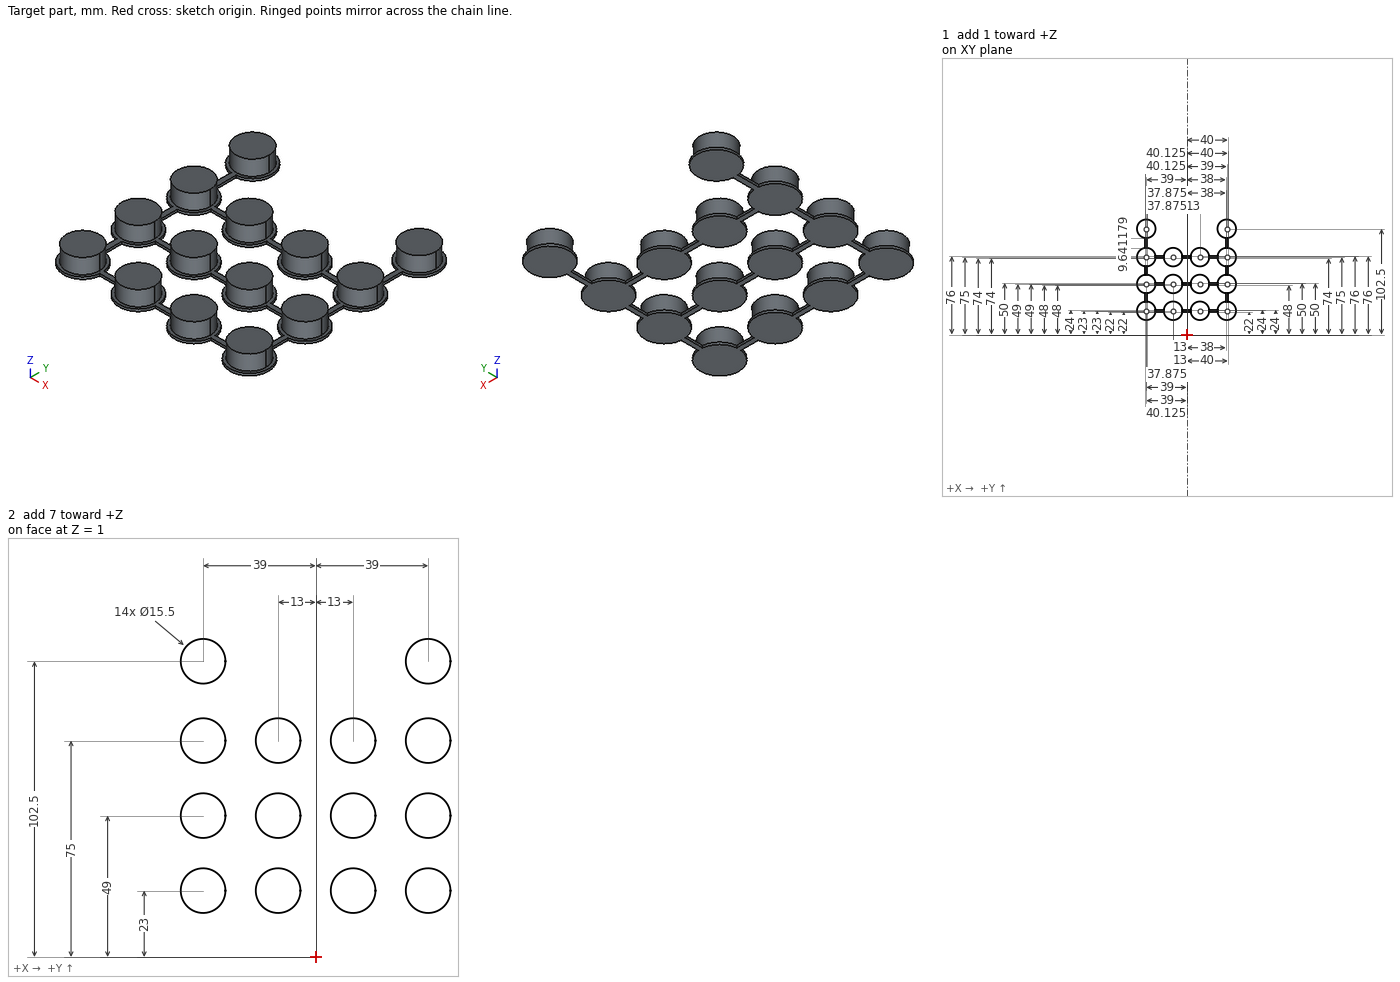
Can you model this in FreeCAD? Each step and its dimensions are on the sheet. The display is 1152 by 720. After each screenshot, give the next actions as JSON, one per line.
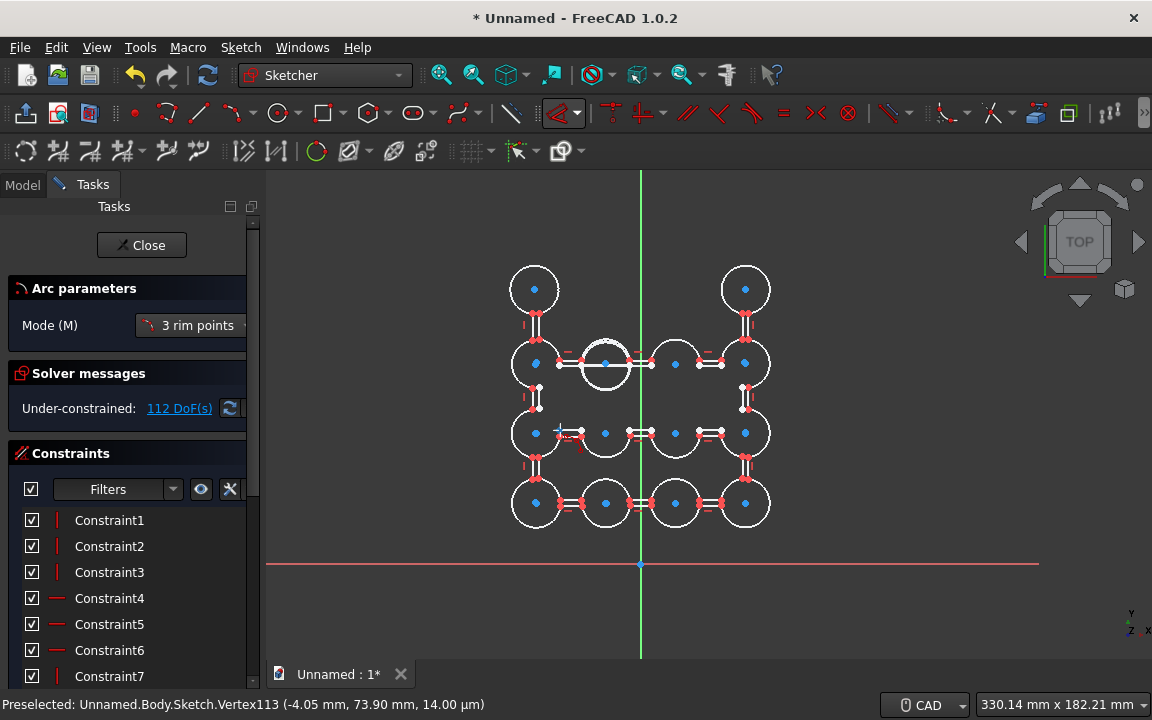
{"action": "left_click", "coordinate": [606, 387]}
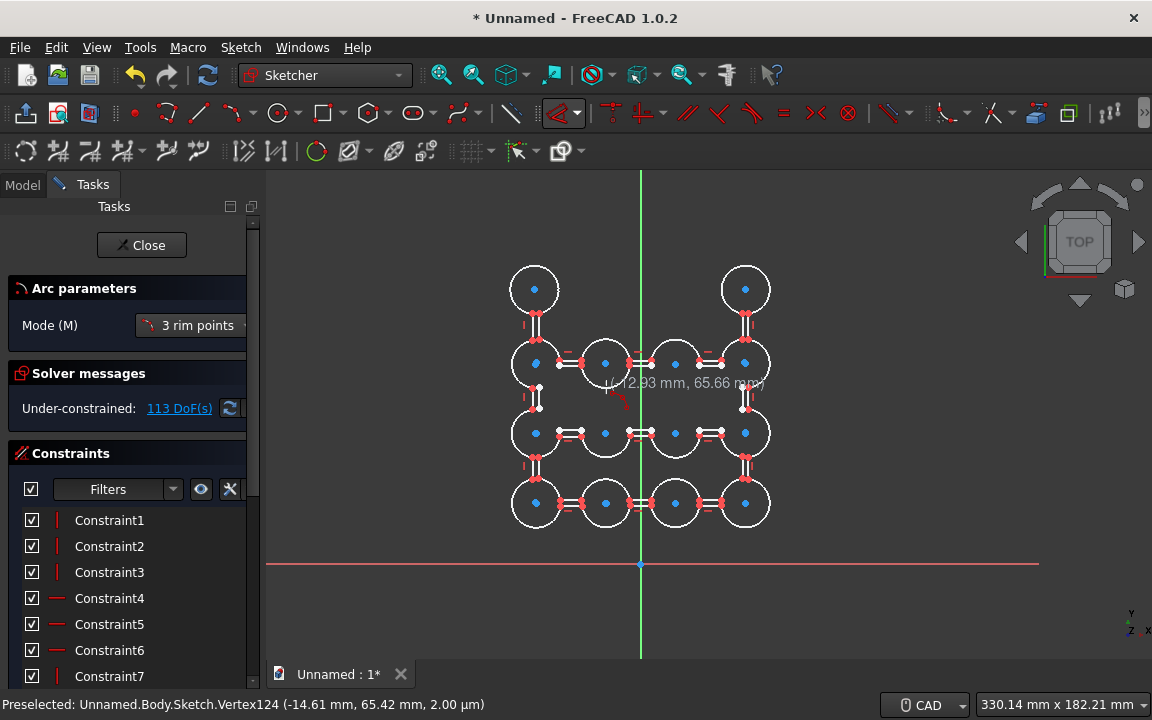
{"action": "scroll", "coordinate": [652, 366], "scroll_direction": "up", "scroll_amount": 6}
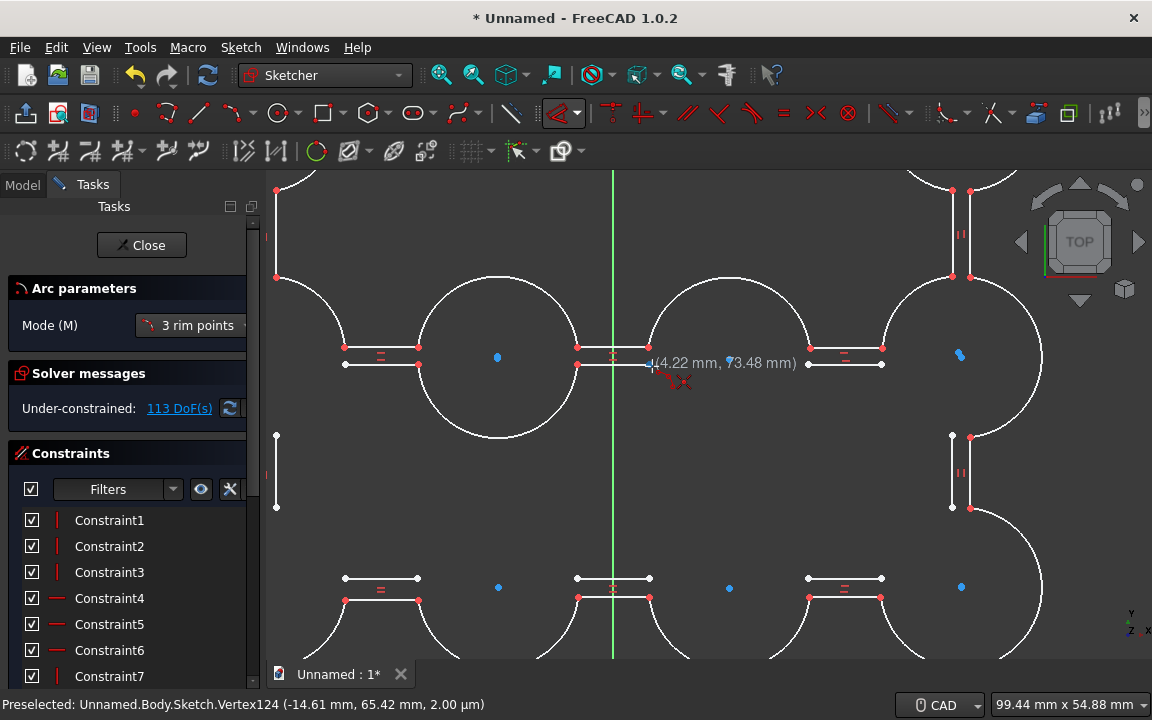
{"action": "left_click", "coordinate": [649, 365]}
{"action": "left_click", "coordinate": [808, 365]}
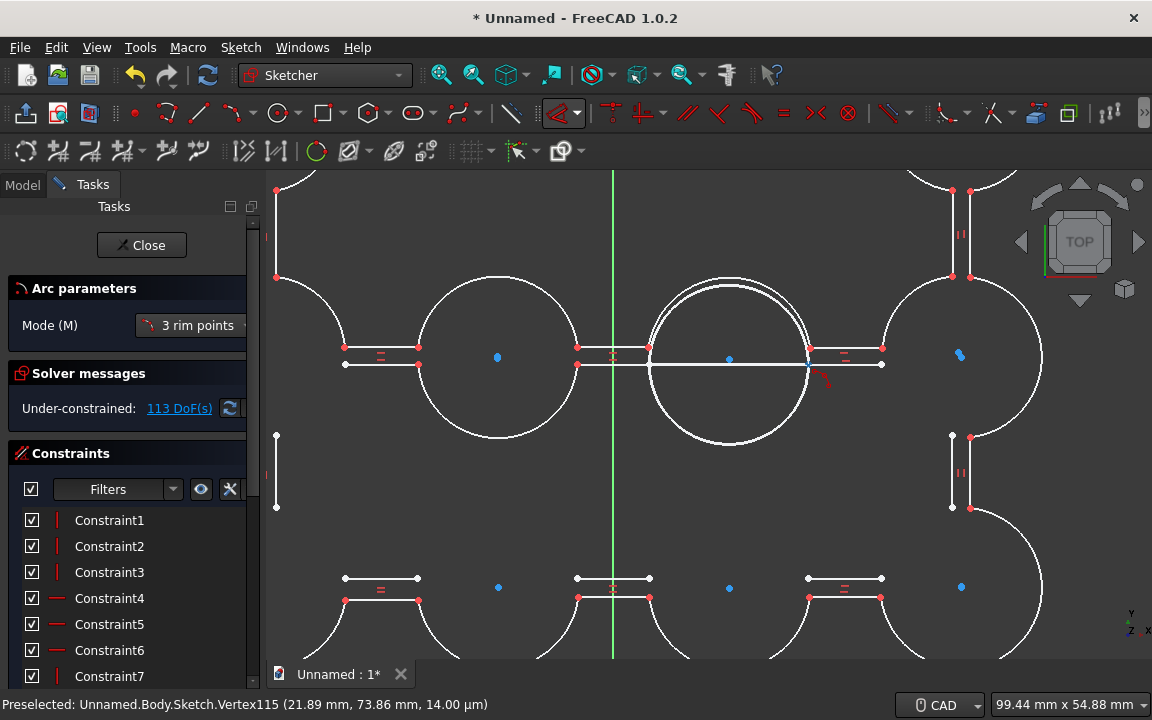
{"action": "scroll", "coordinate": [652, 366], "scroll_direction": "down", "scroll_amount": 6}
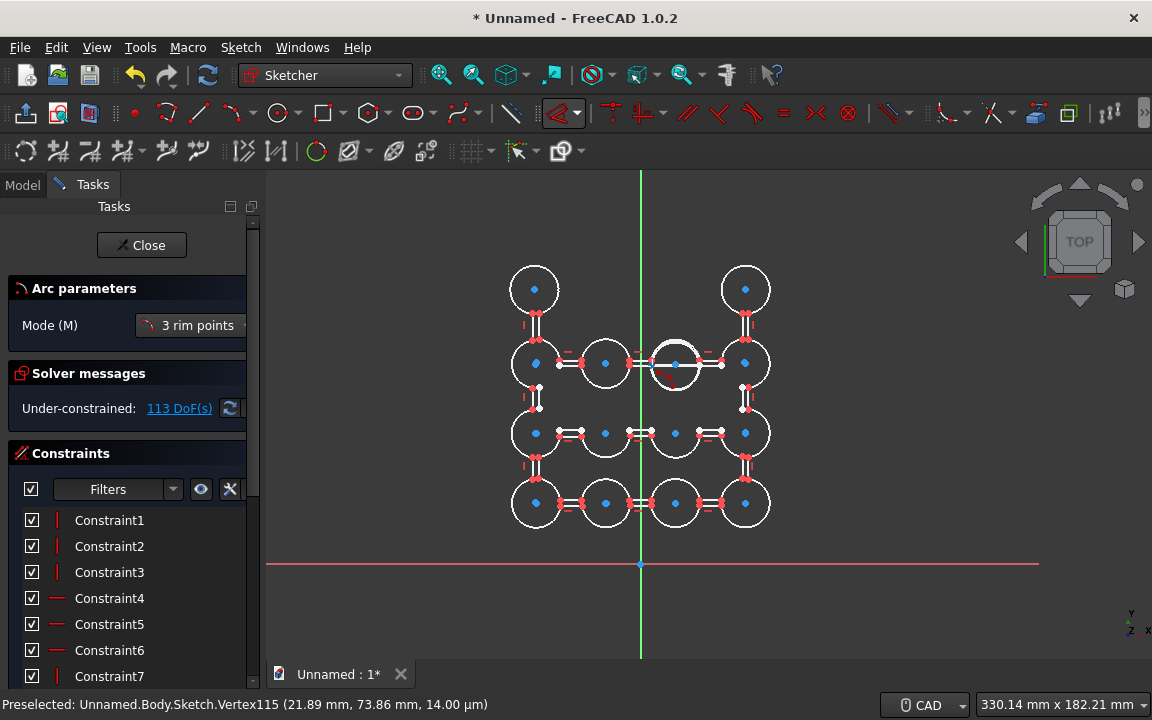
{"action": "left_click", "coordinate": [676, 387]}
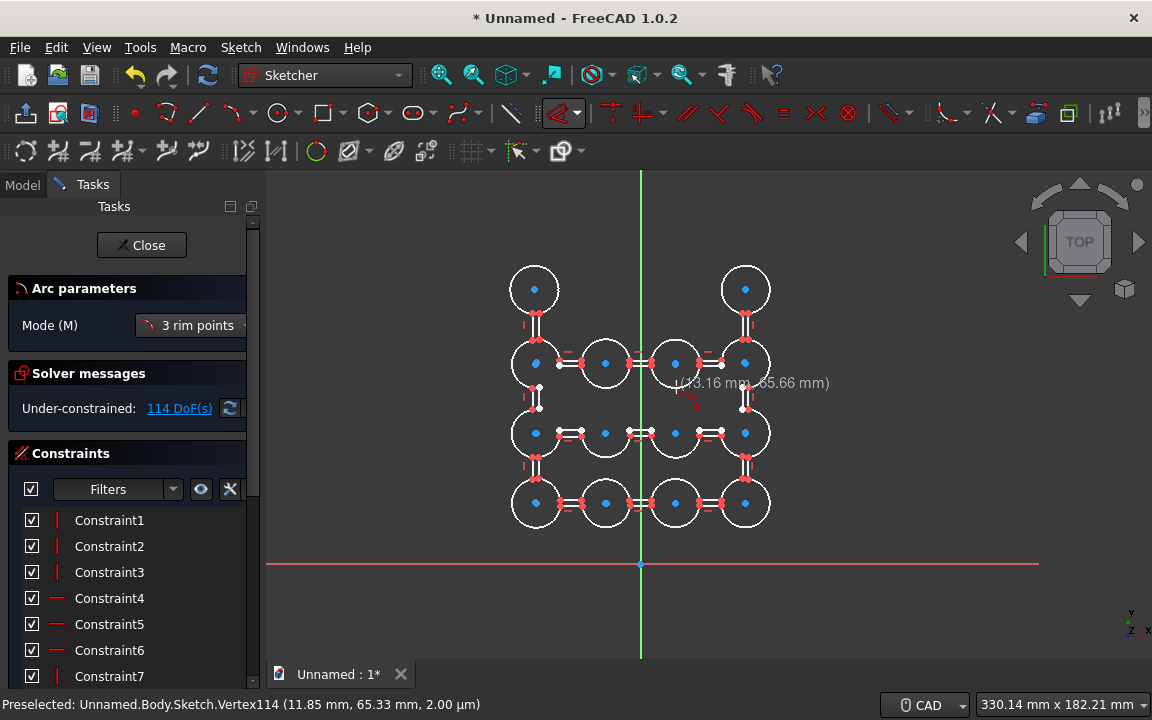
{"action": "scroll", "coordinate": [721, 366], "scroll_direction": "up", "scroll_amount": 6}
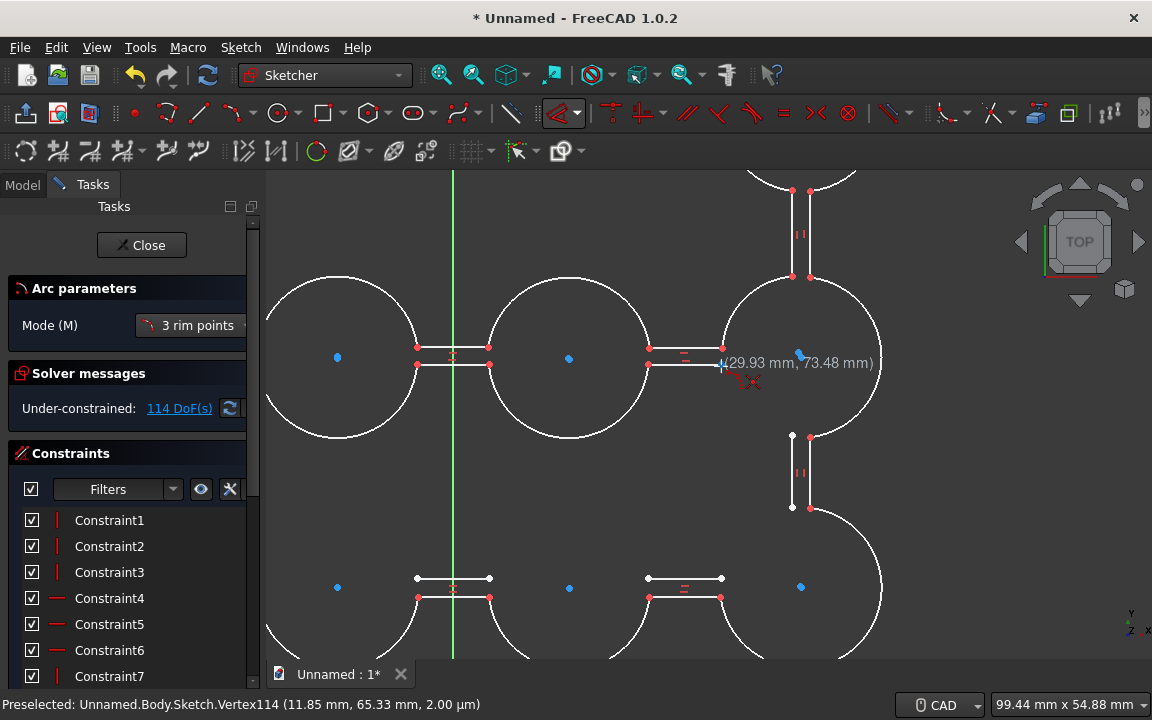
{"action": "left_click", "coordinate": [721, 365]}
{"action": "left_click", "coordinate": [792, 436]}
{"action": "left_click", "coordinate": [744, 412]}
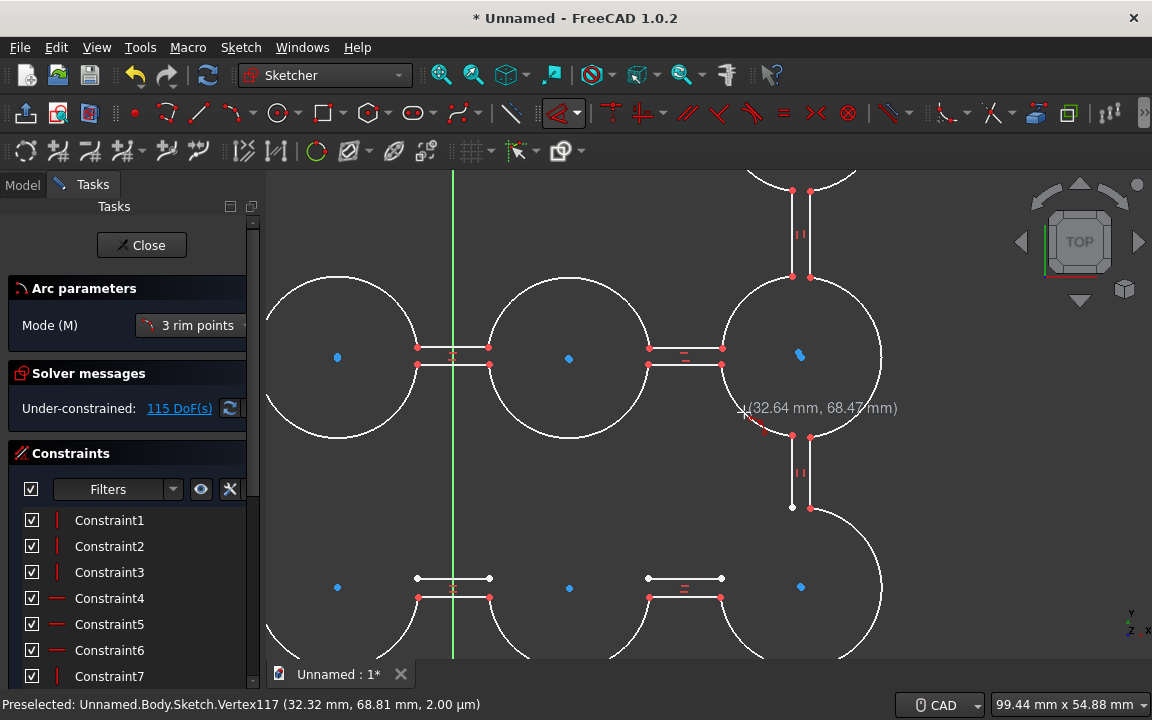
{"action": "left_click", "coordinate": [792, 508]}
{"action": "left_click", "coordinate": [721, 579]}
{"action": "left_click", "coordinate": [744, 530]}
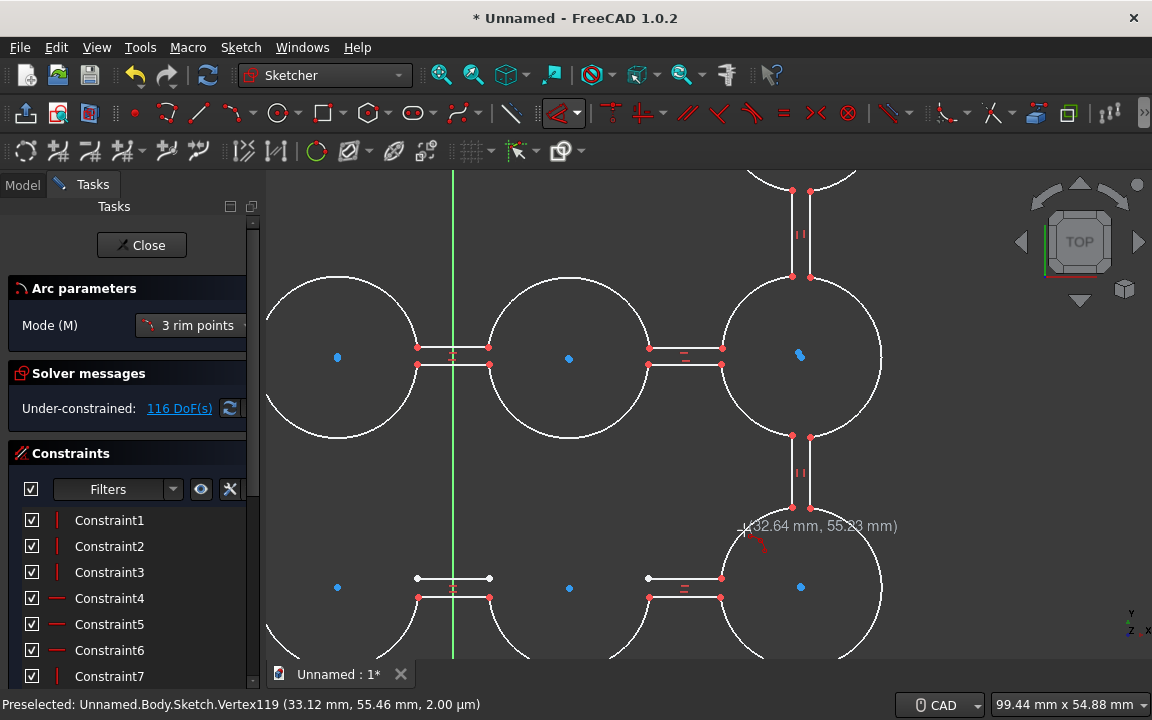
{"action": "left_click", "coordinate": [648, 579]}
{"action": "left_click", "coordinate": [489, 579]}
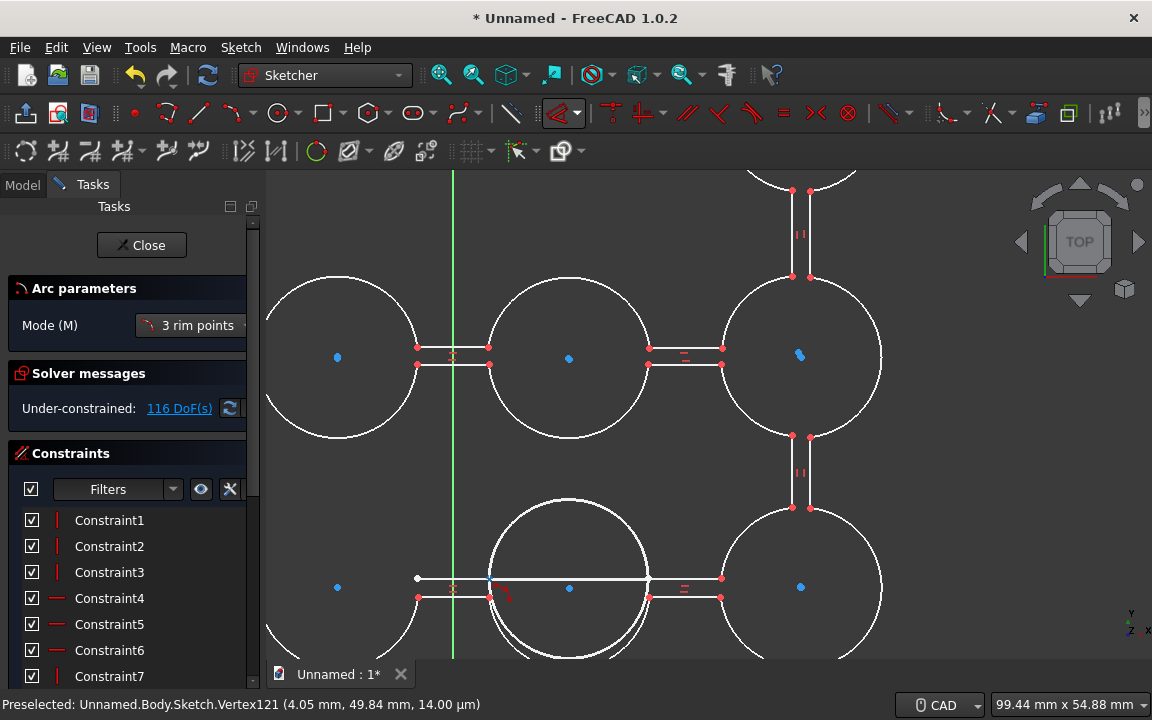
{"action": "scroll", "coordinate": [721, 366], "scroll_direction": "down", "scroll_amount": 6}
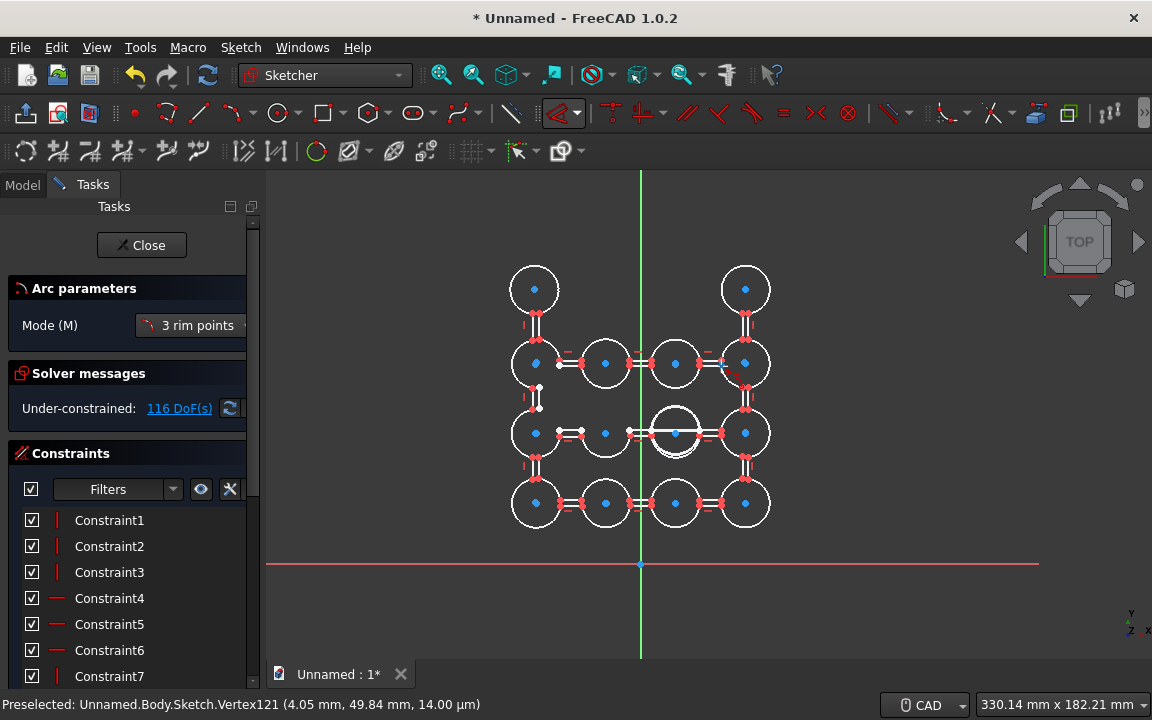
{"action": "left_click", "coordinate": [676, 409]}